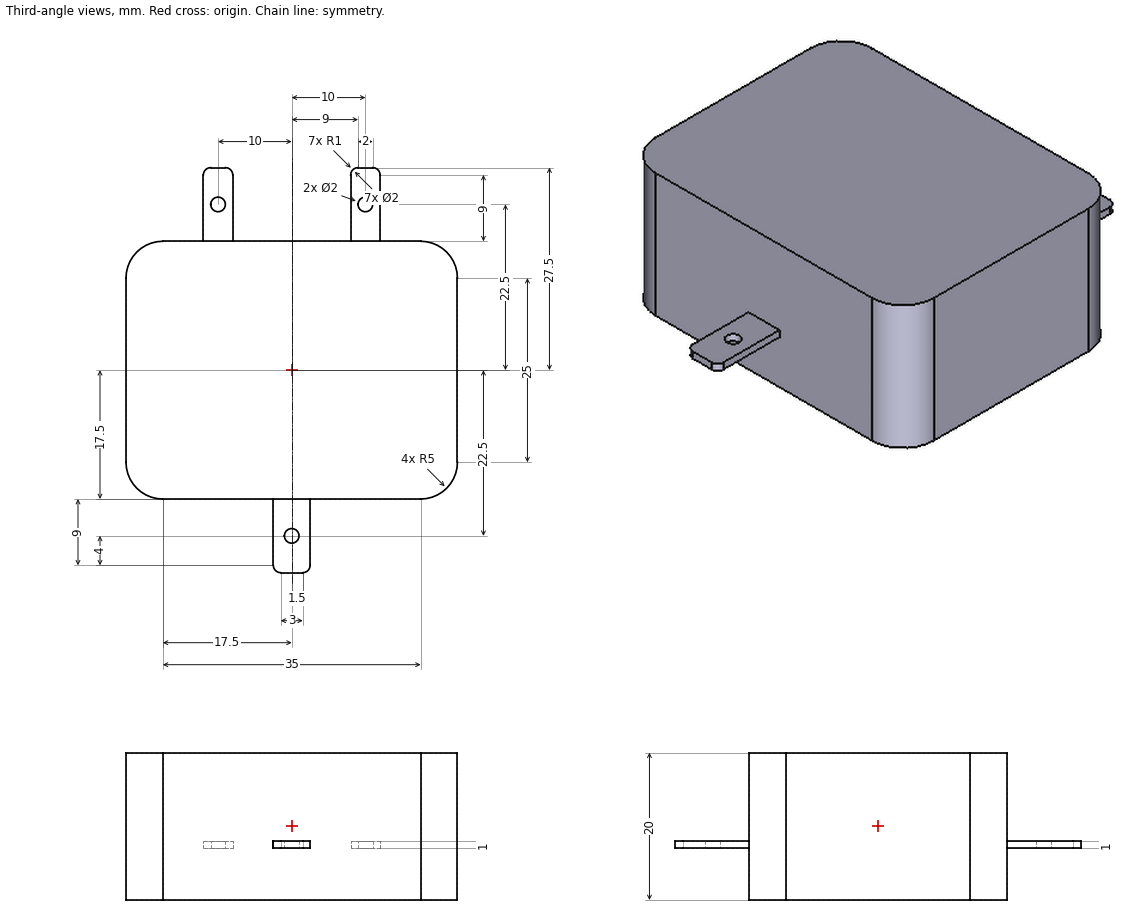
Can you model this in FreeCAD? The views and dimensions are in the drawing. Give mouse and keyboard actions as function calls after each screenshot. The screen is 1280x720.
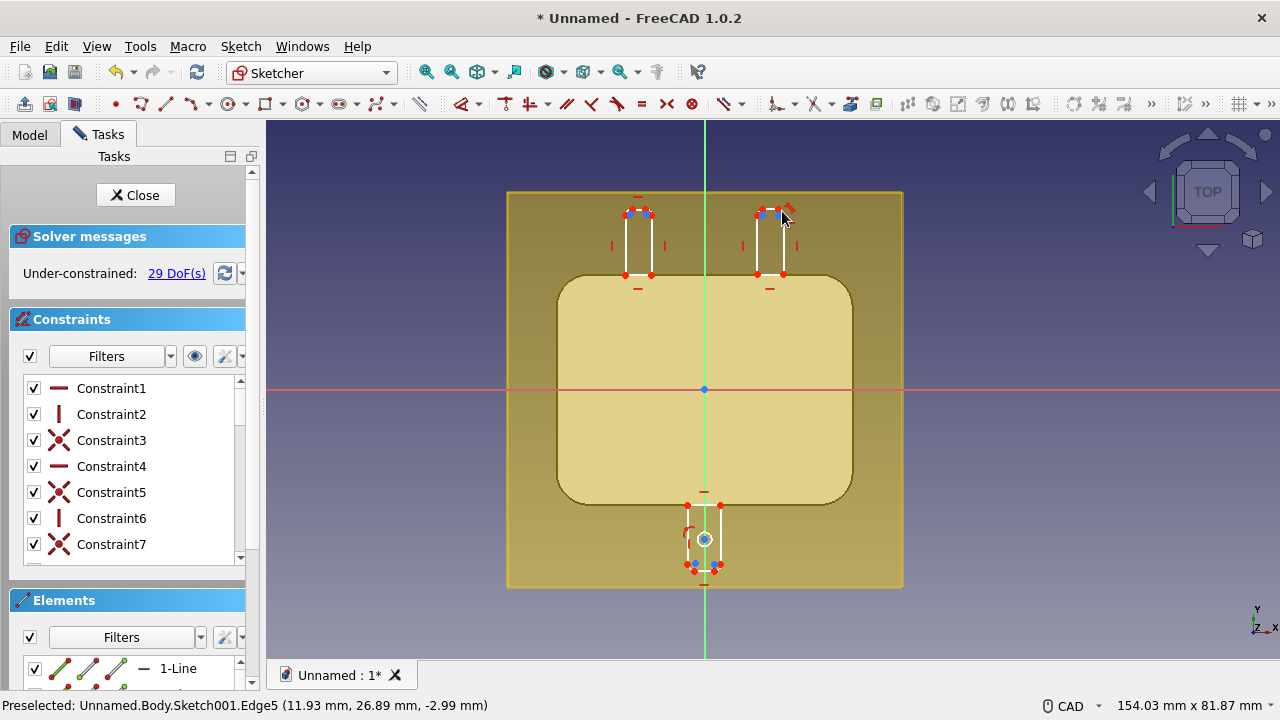
click(757, 257)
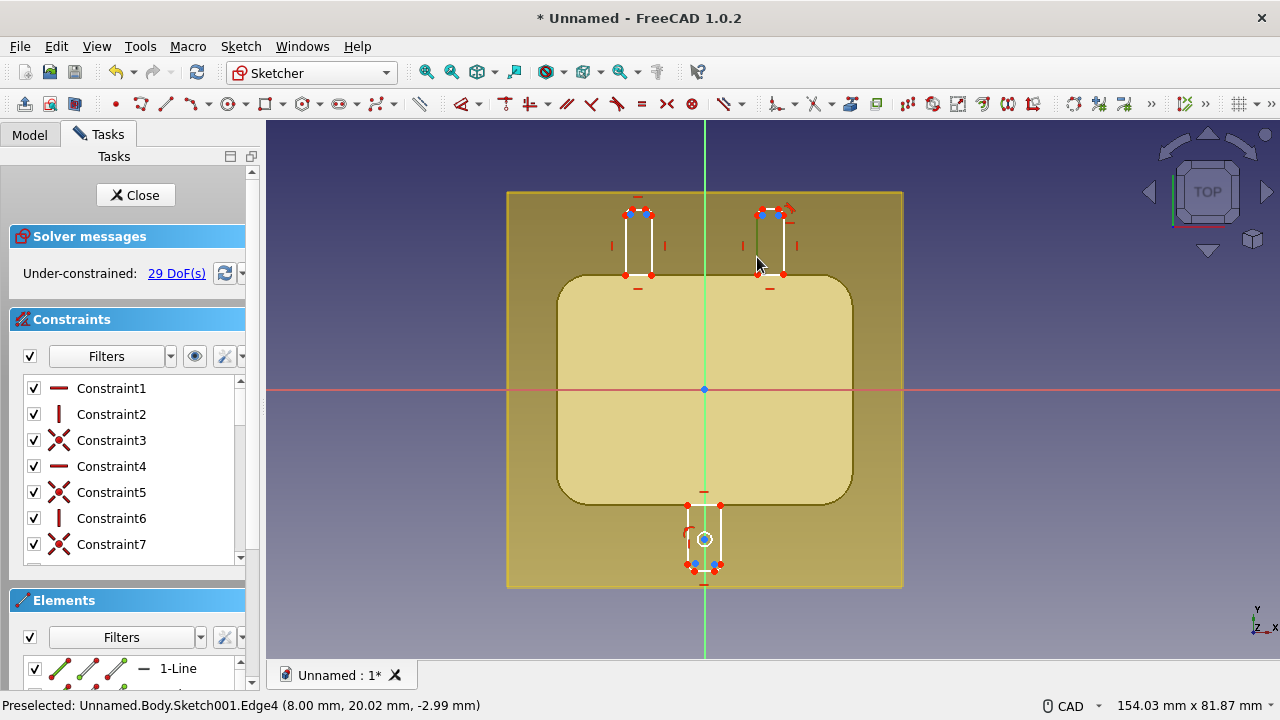
scroll(759, 211, up, 6)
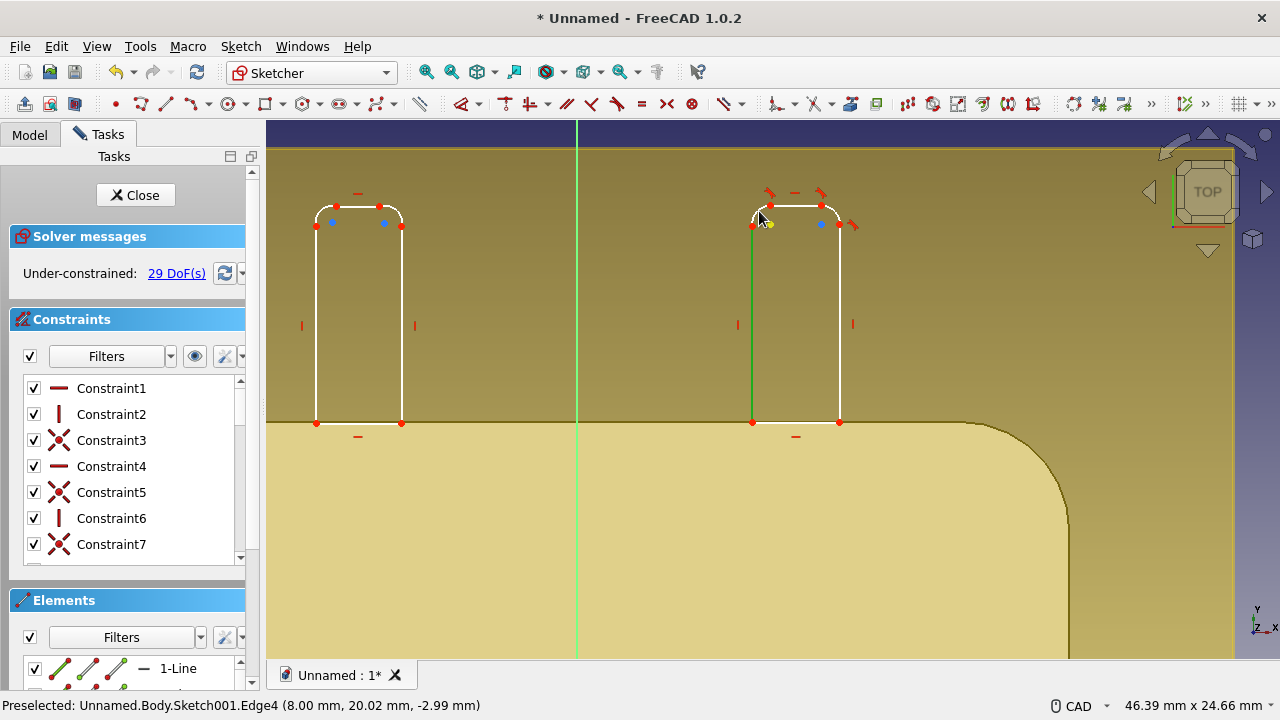
click(757, 212)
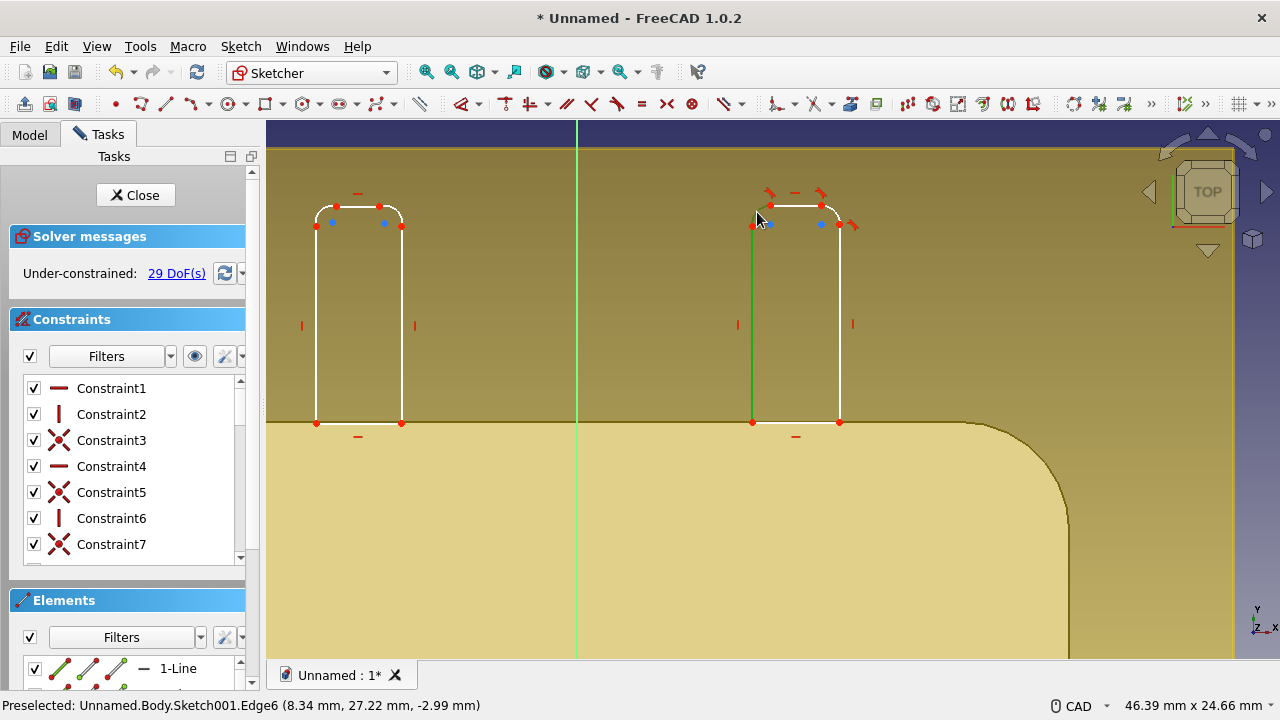
click(617, 104)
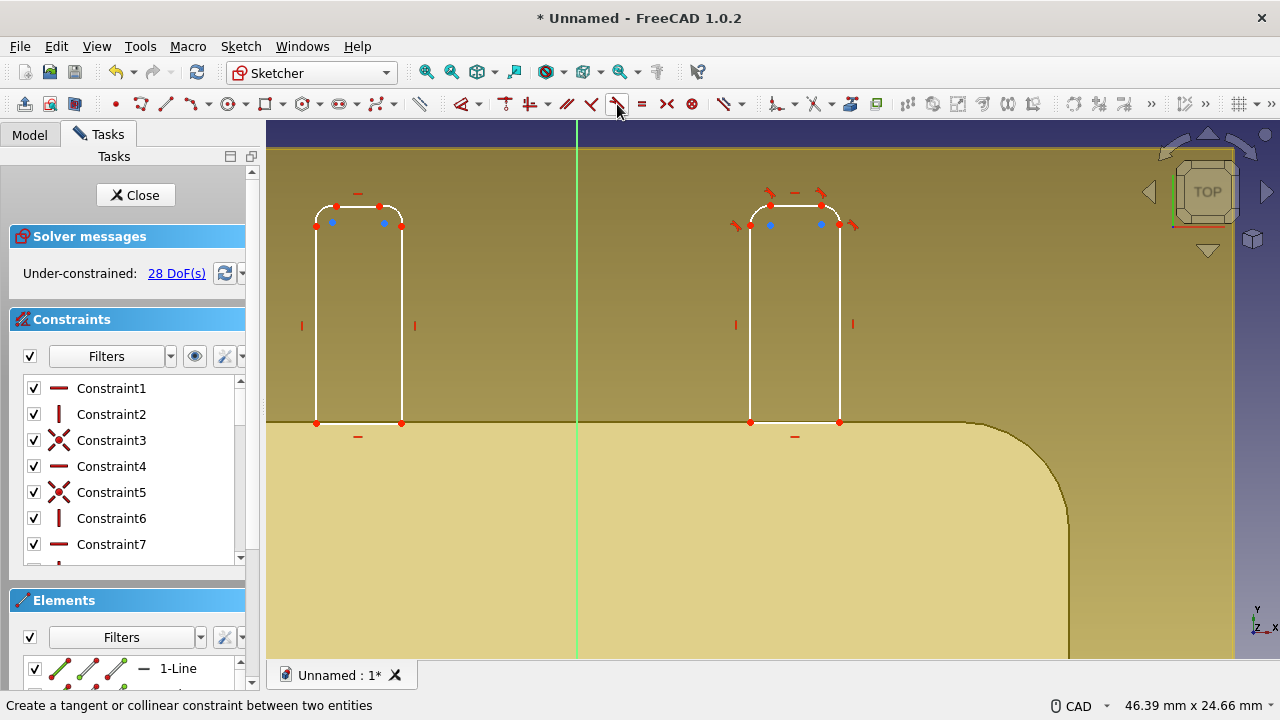
click(350, 207)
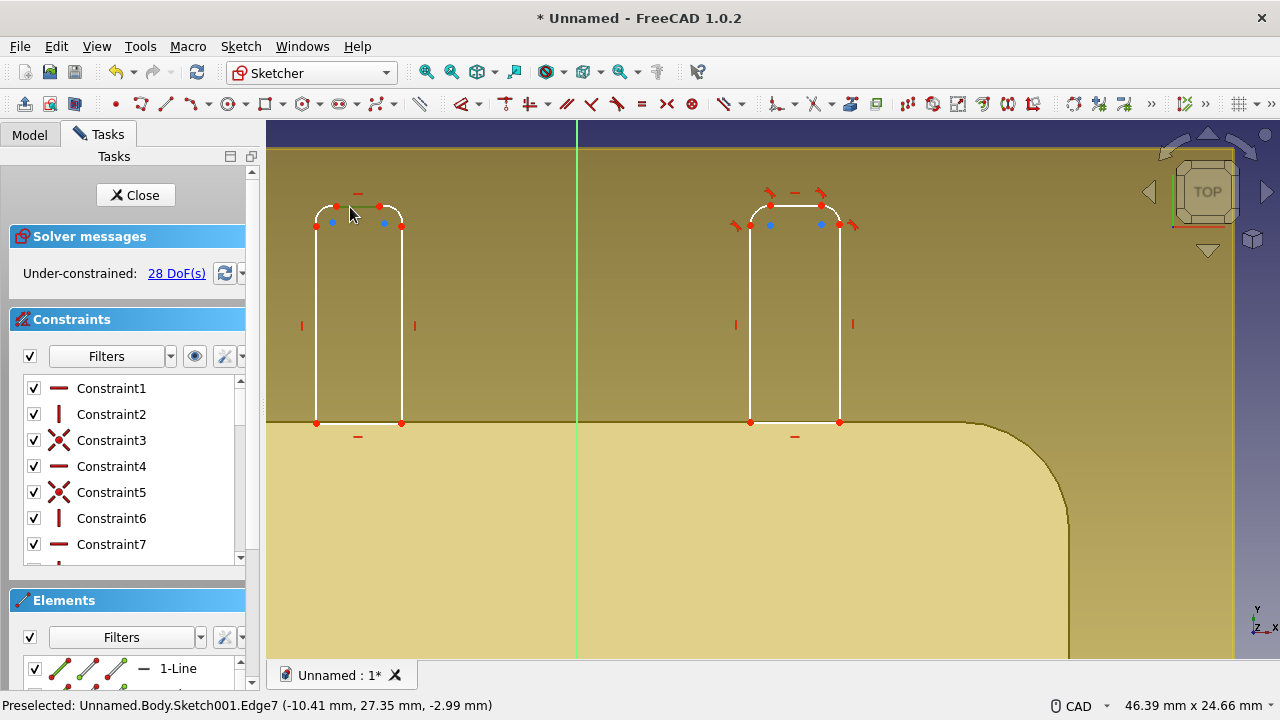
scroll(401, 216, up, 2)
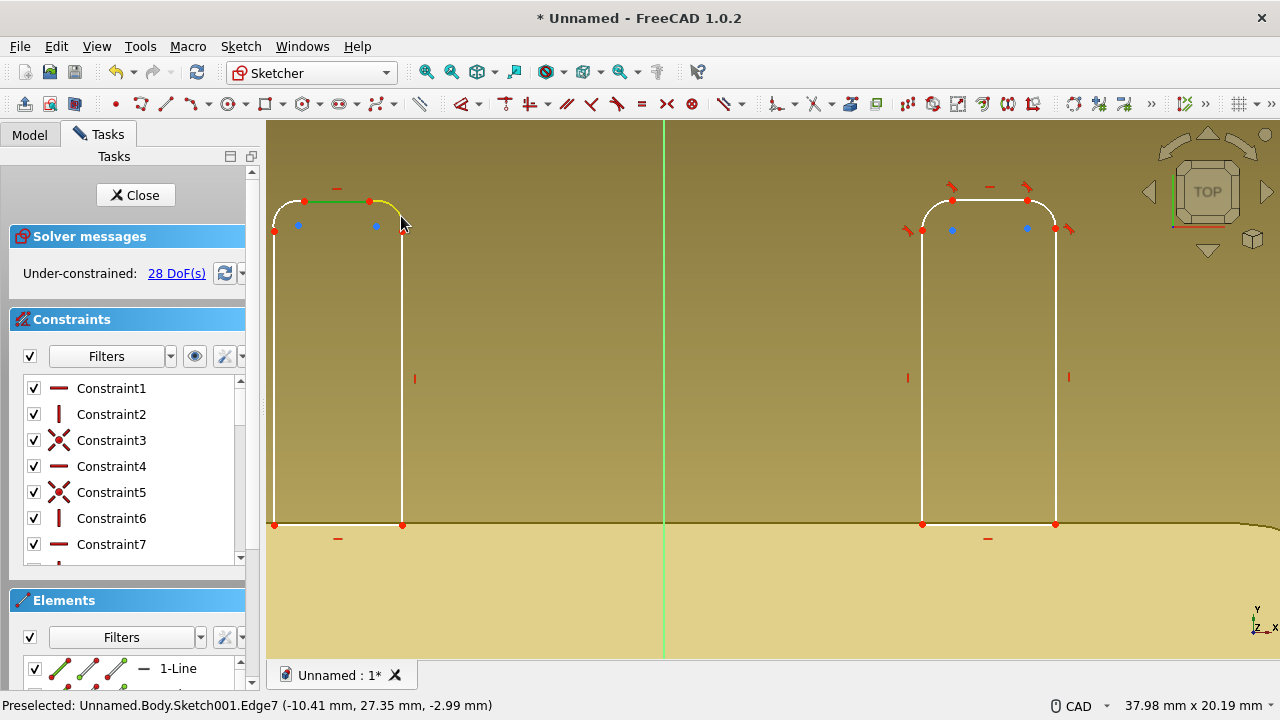
click(400, 216)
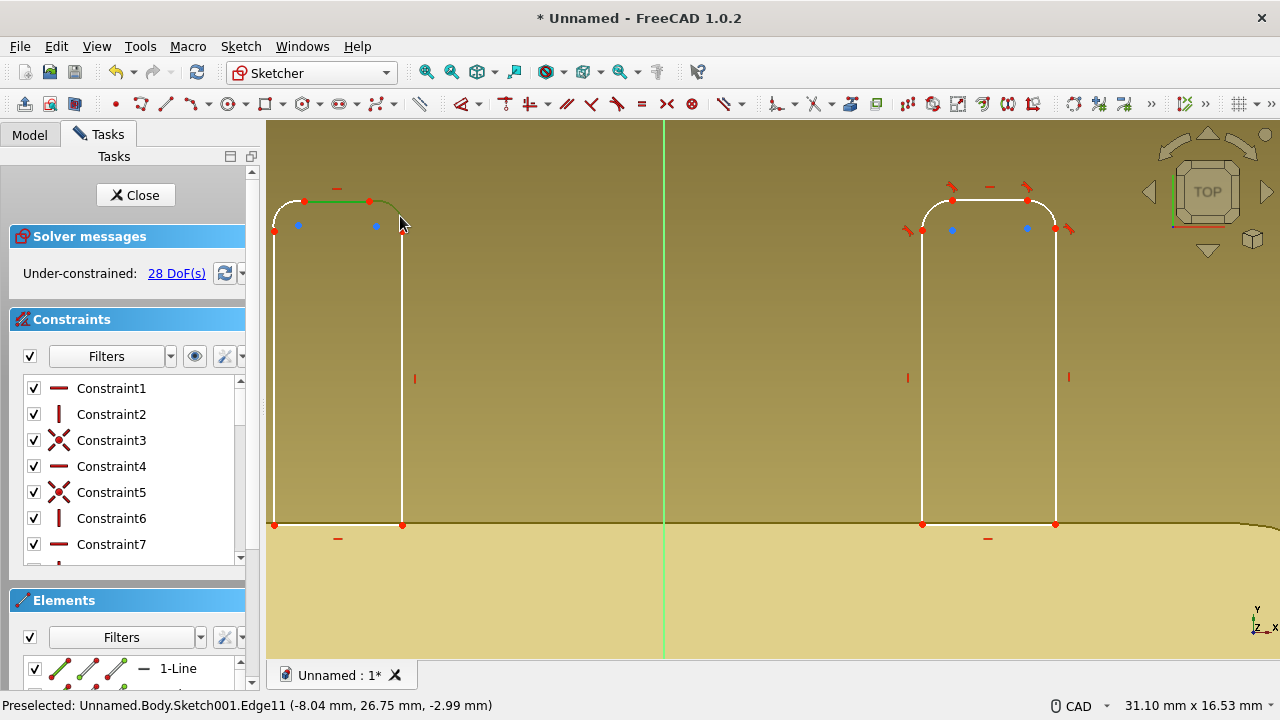
click(617, 104)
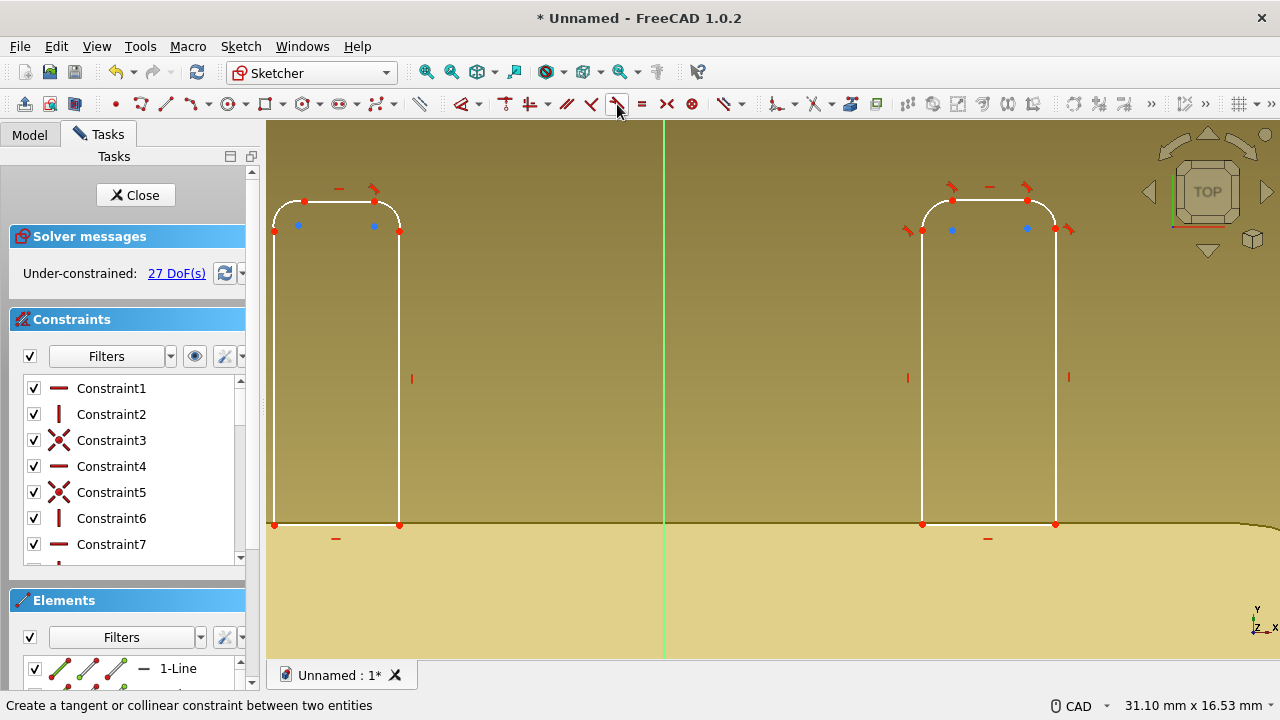
click(326, 202)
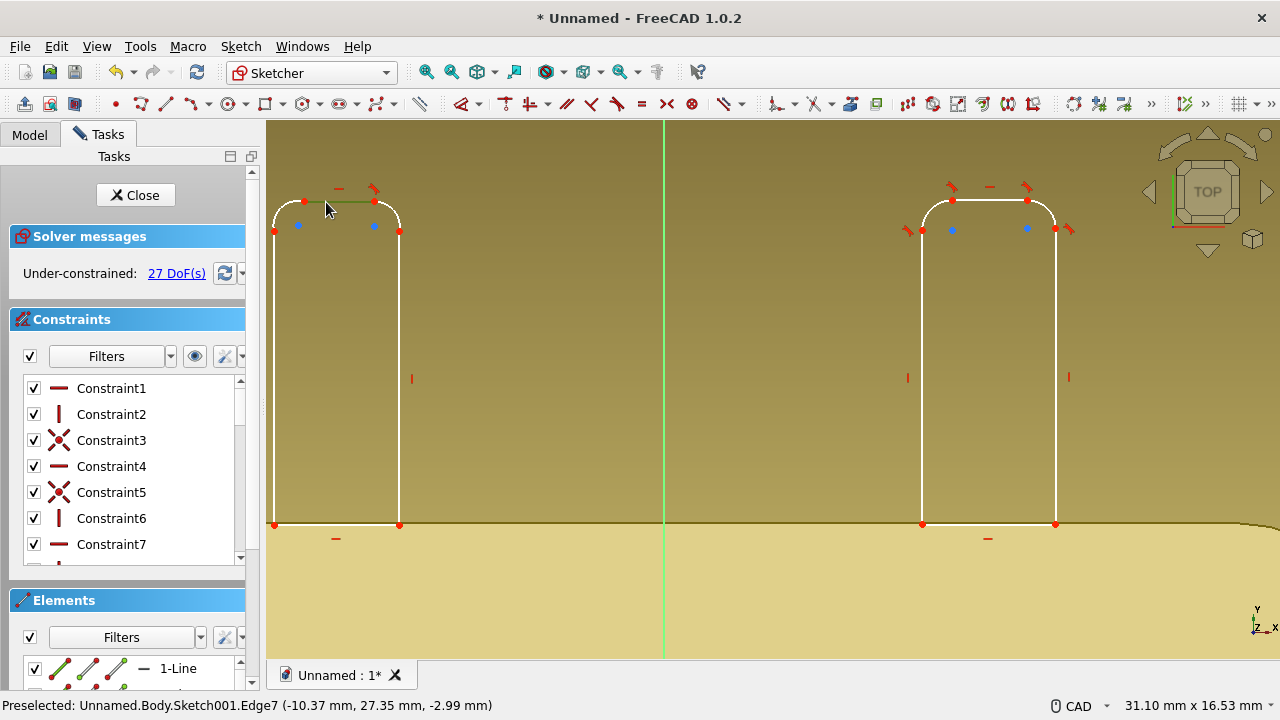
scroll(295, 201, up, 2)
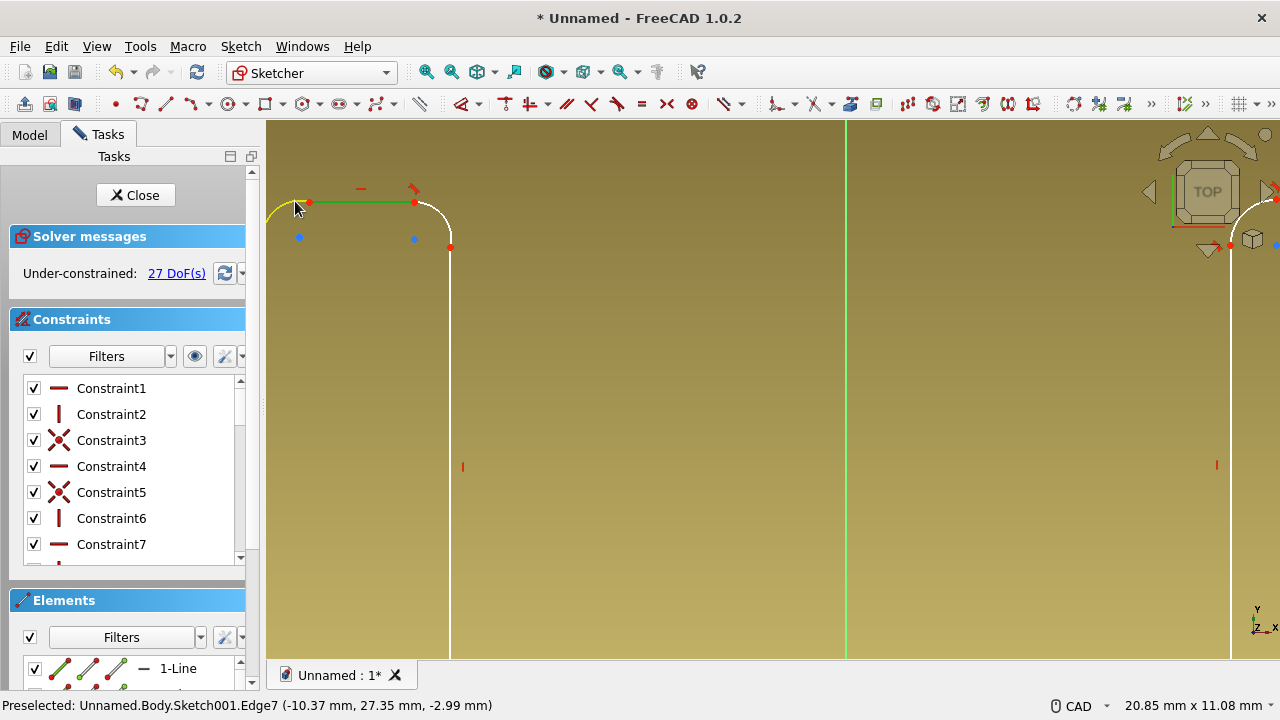
click(294, 201)